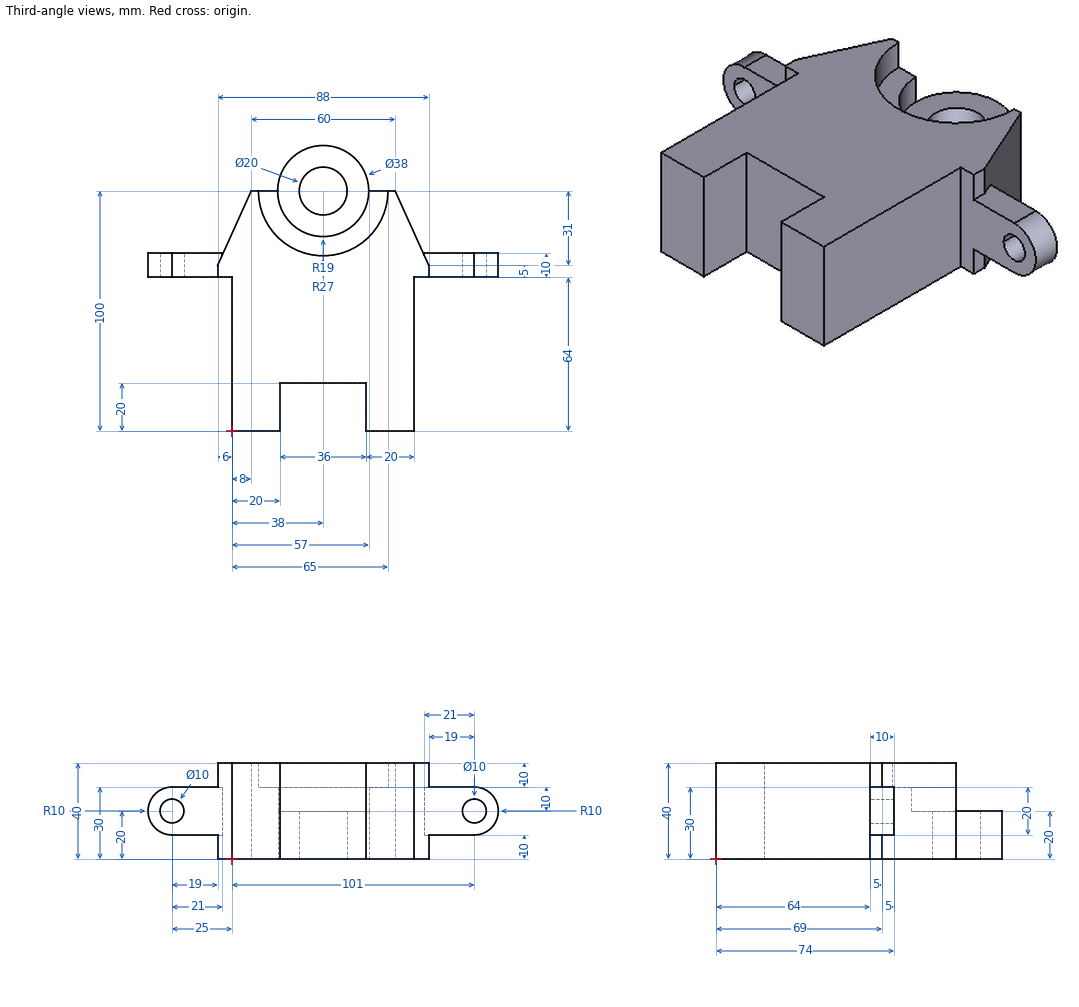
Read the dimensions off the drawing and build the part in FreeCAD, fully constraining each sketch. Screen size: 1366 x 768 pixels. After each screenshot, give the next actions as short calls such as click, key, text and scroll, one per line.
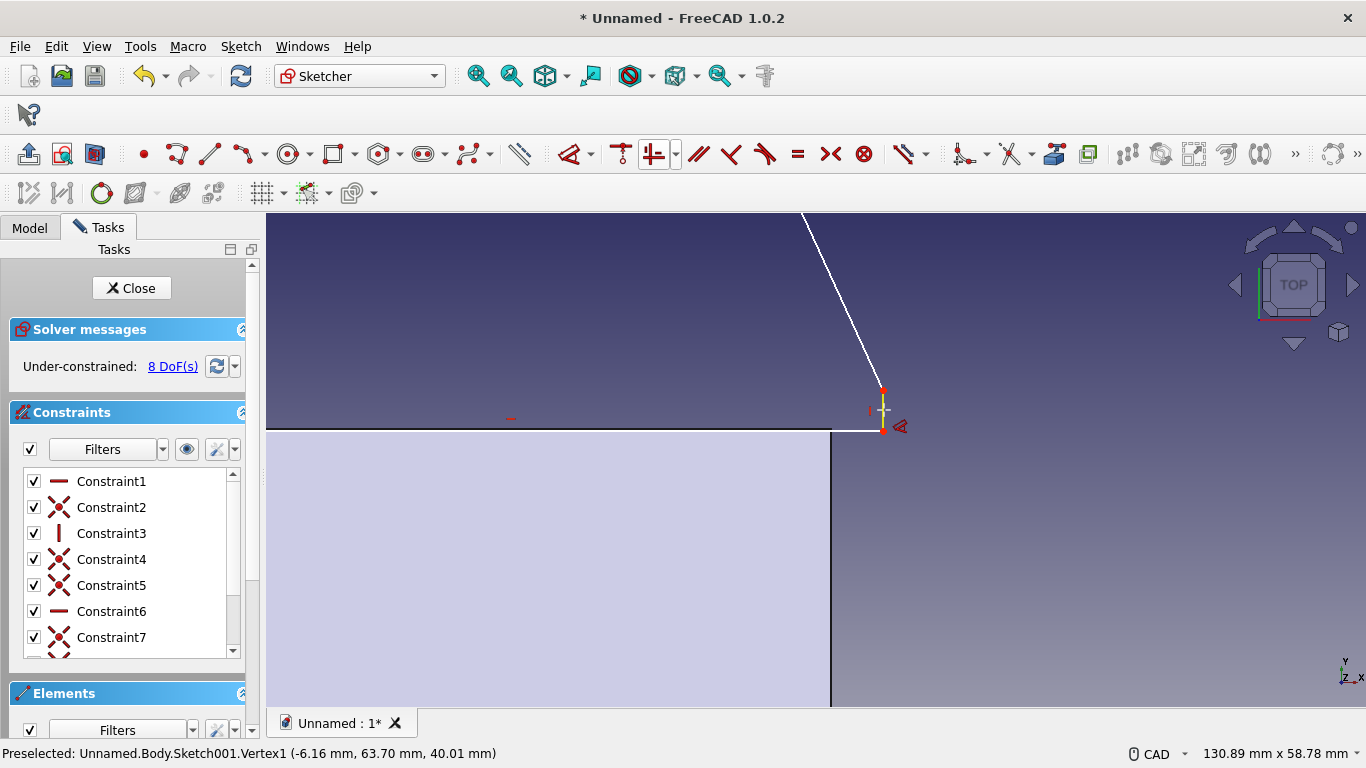
click(883, 411)
click(917, 411)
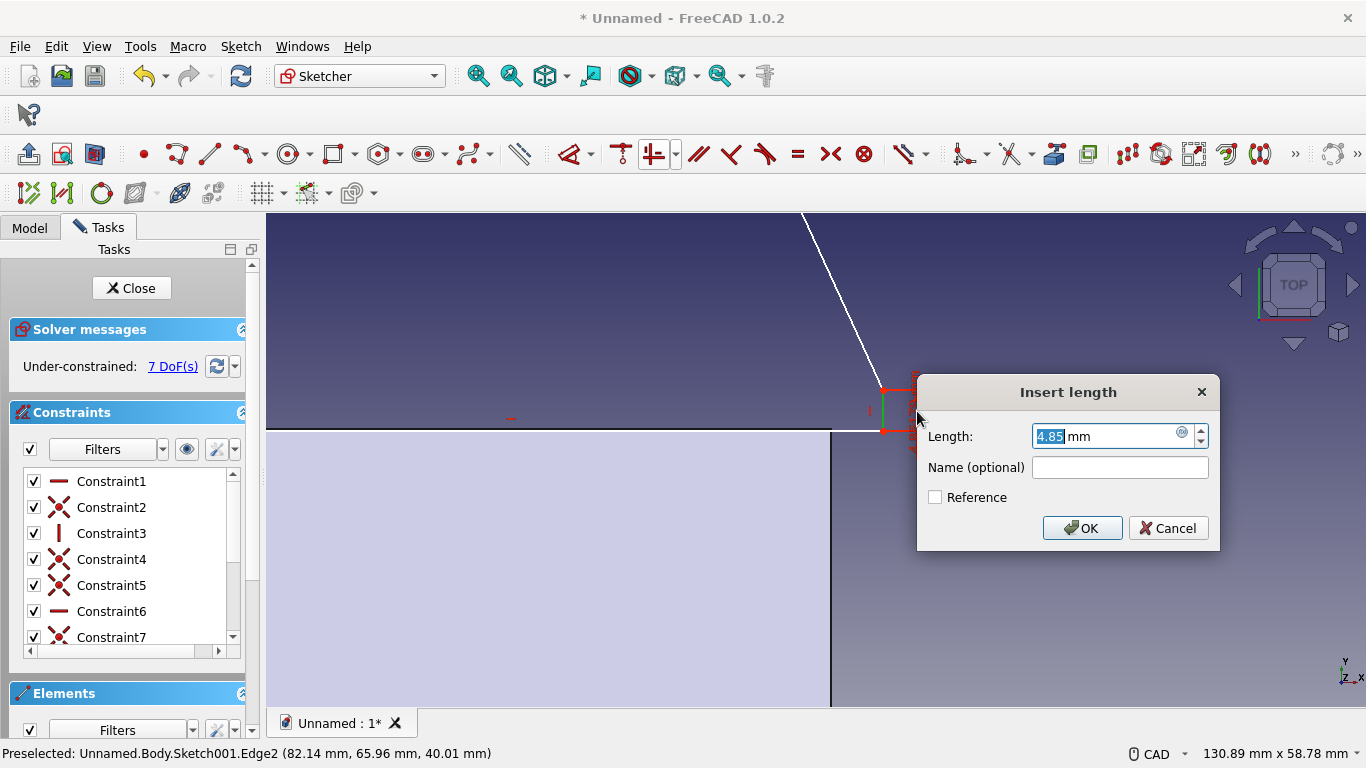
text(5)
key(Return)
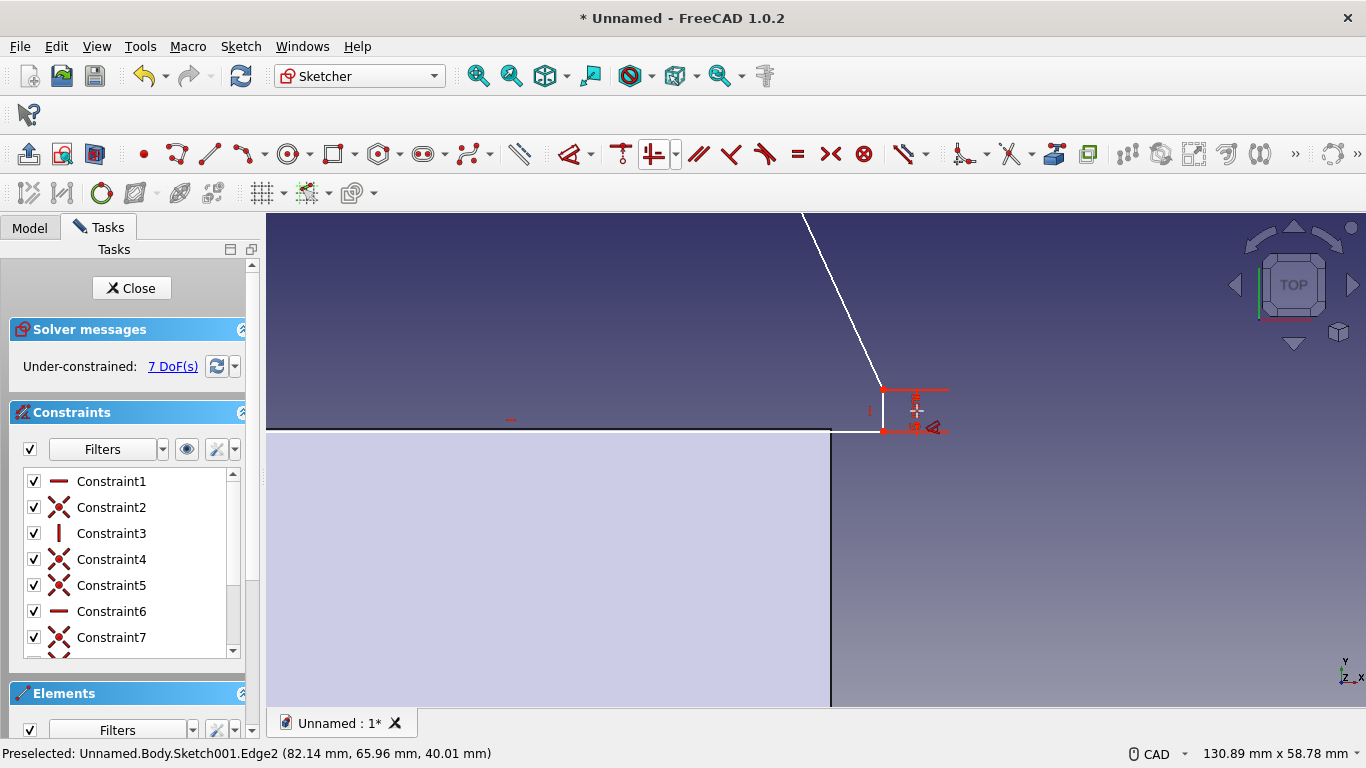
scroll(885, 410, down, 5)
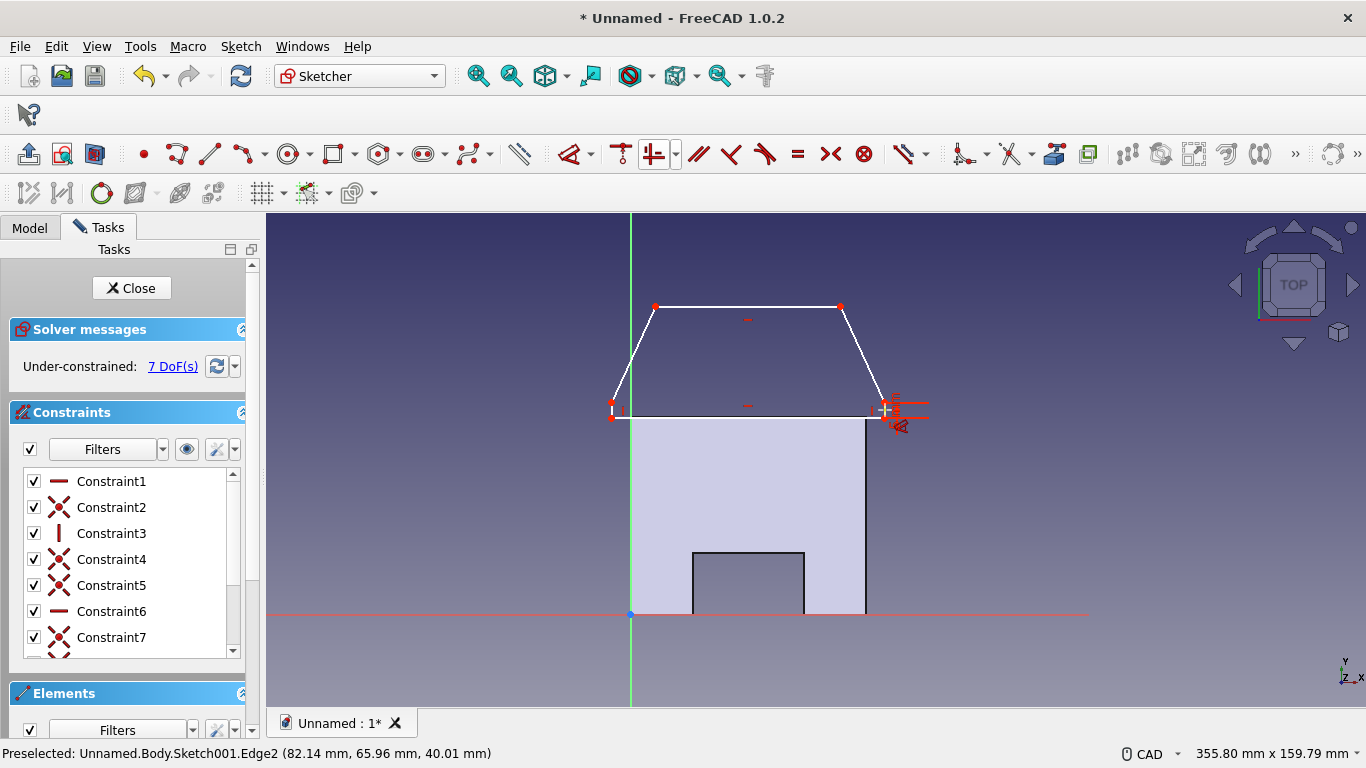
scroll(612, 408, up, 6)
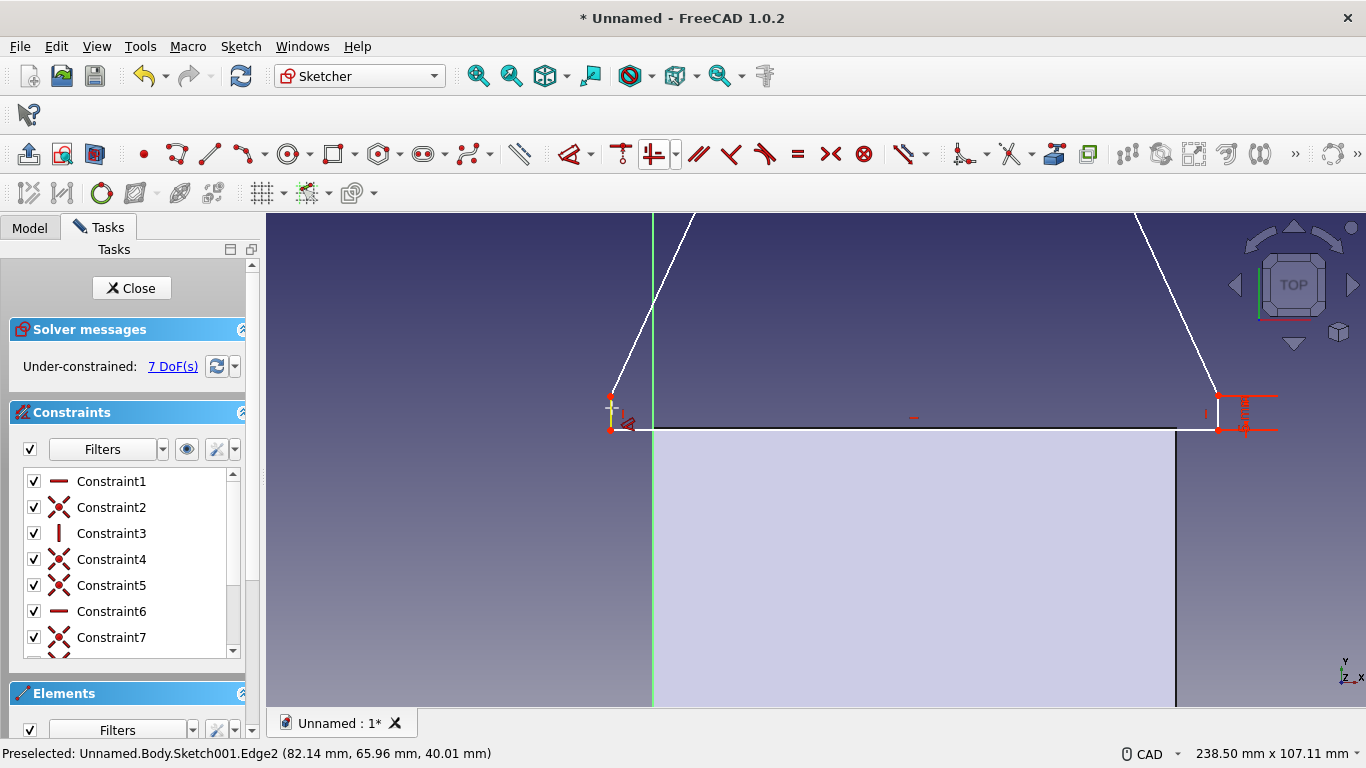
click(610, 406)
click(576, 416)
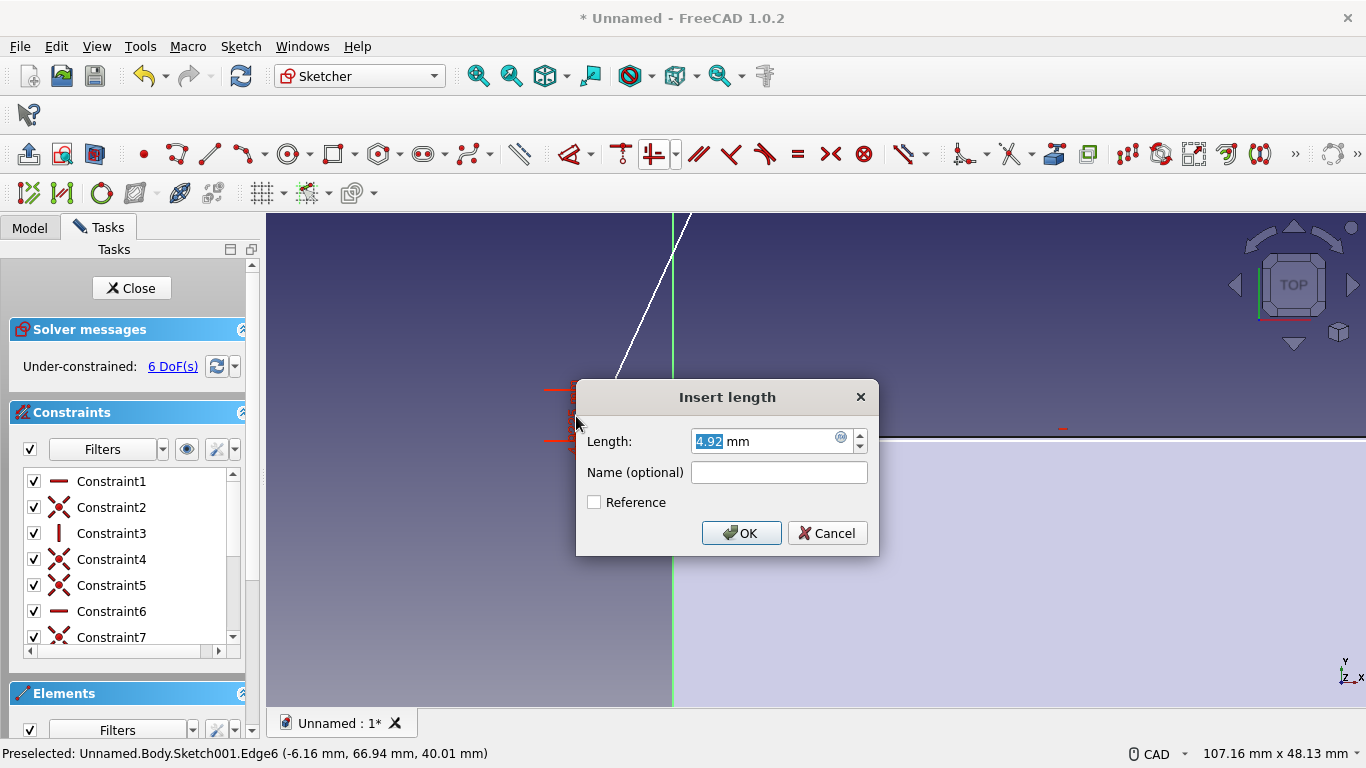
text(5)
key(Return)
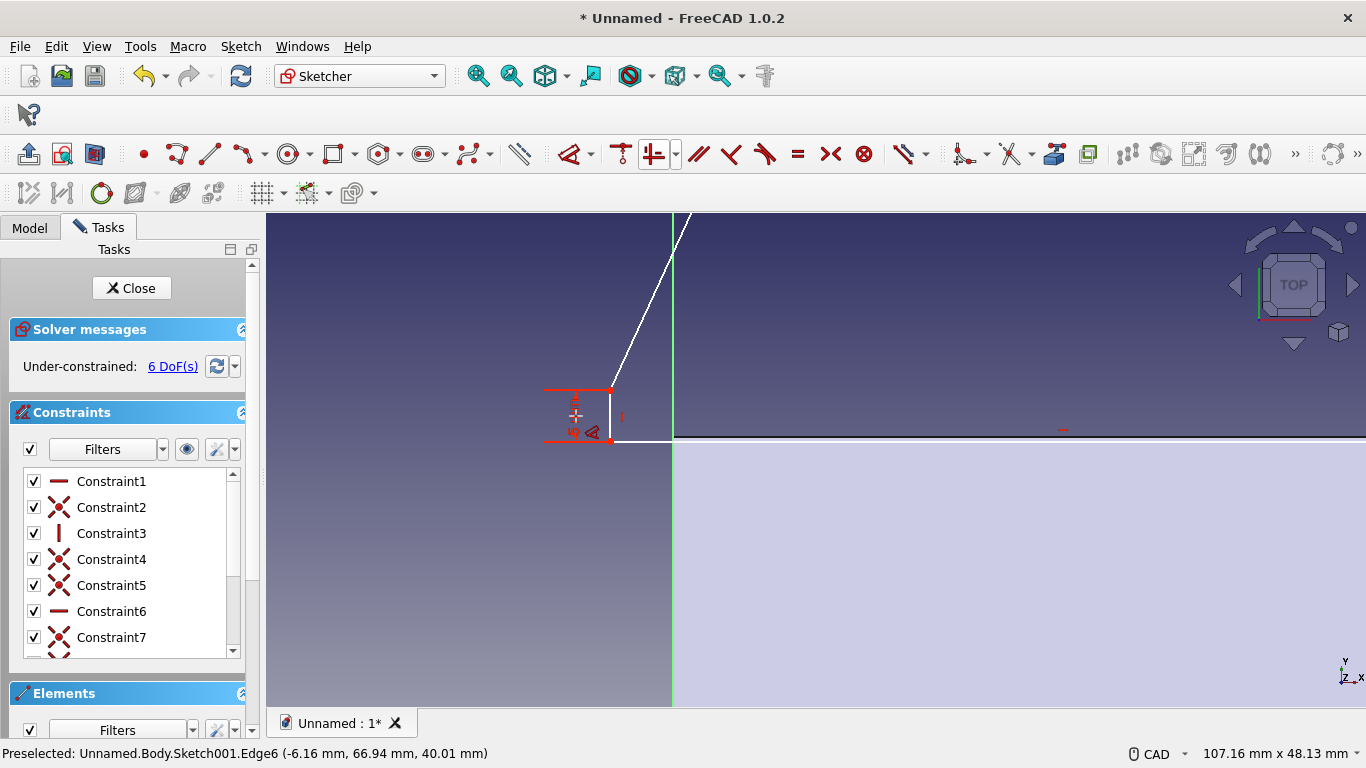
click(882, 442)
click(906, 408)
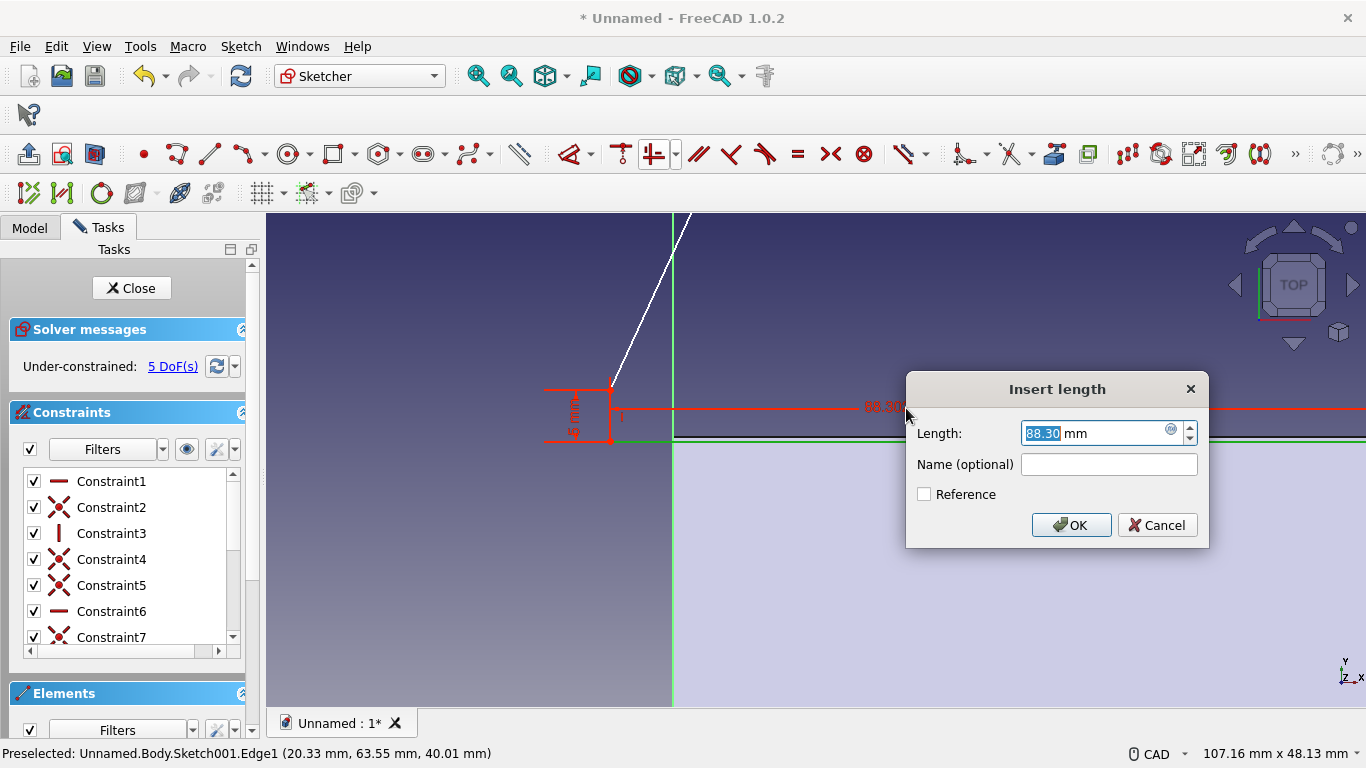
text(88)
key(Return)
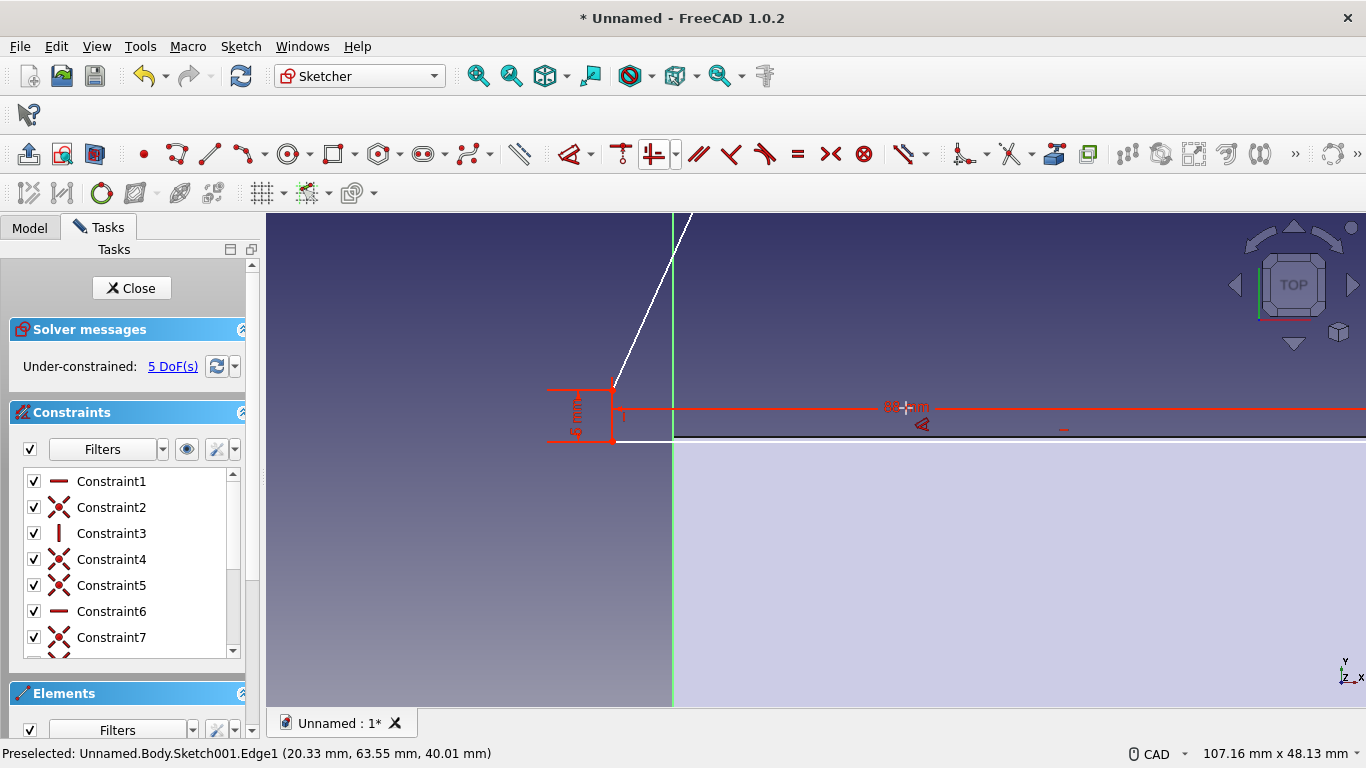
scroll(611, 408, down, 6)